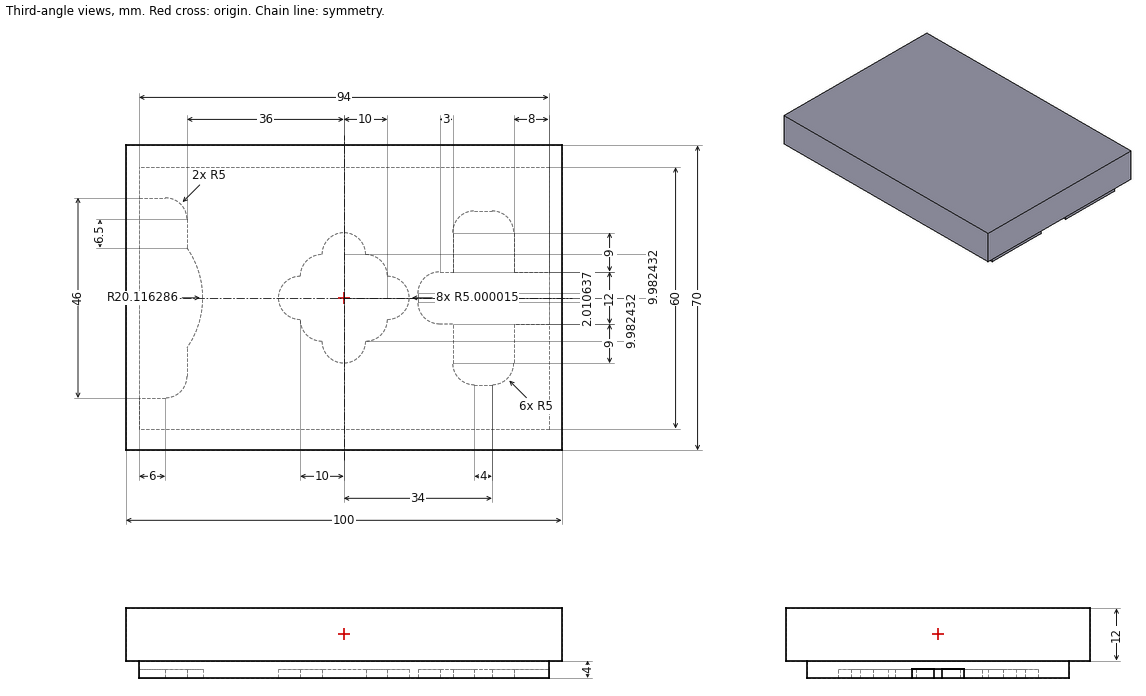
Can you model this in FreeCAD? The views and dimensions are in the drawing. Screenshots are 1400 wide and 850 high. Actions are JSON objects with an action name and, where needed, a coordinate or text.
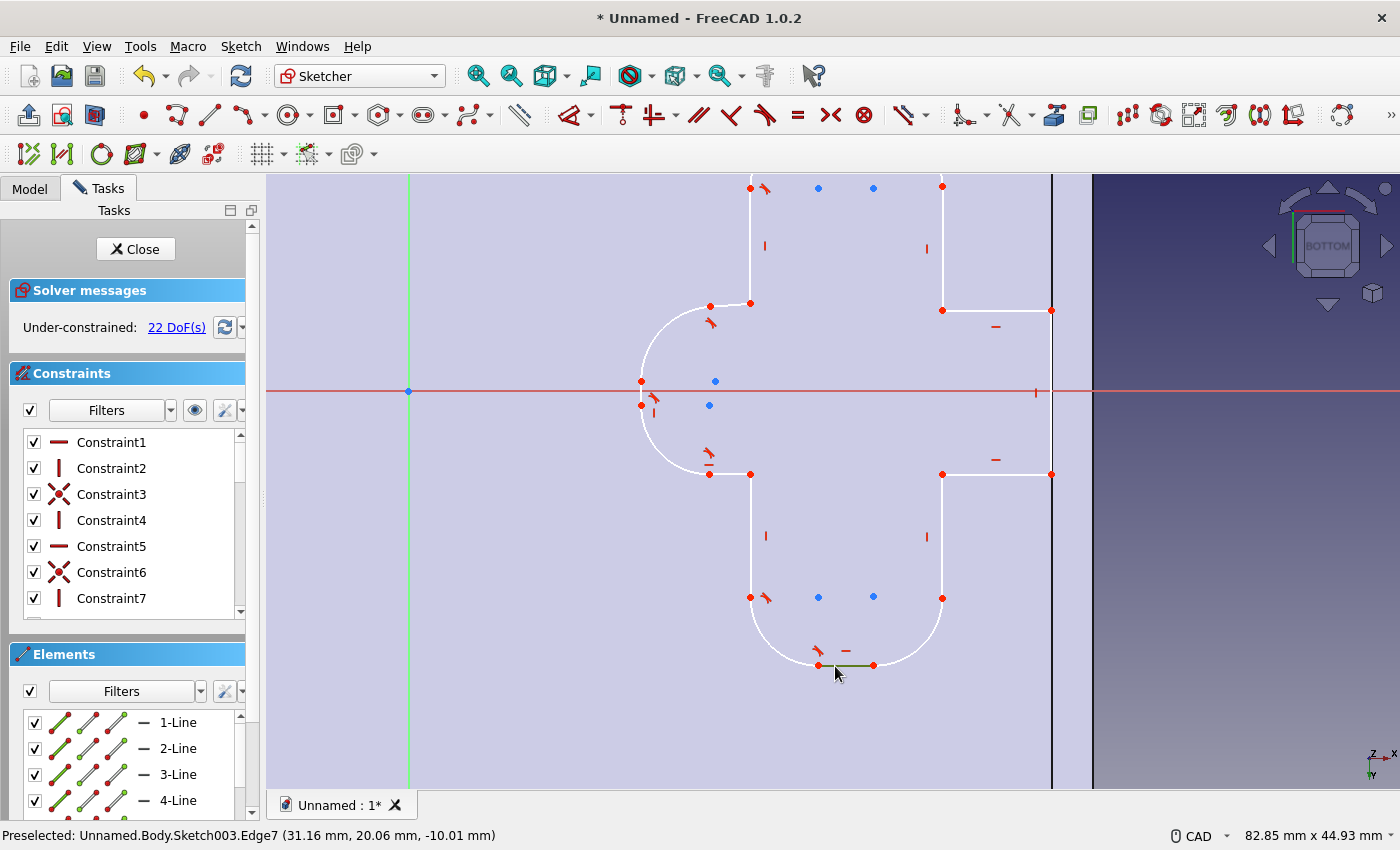
{"action": "left_click", "coordinate": [905, 658]}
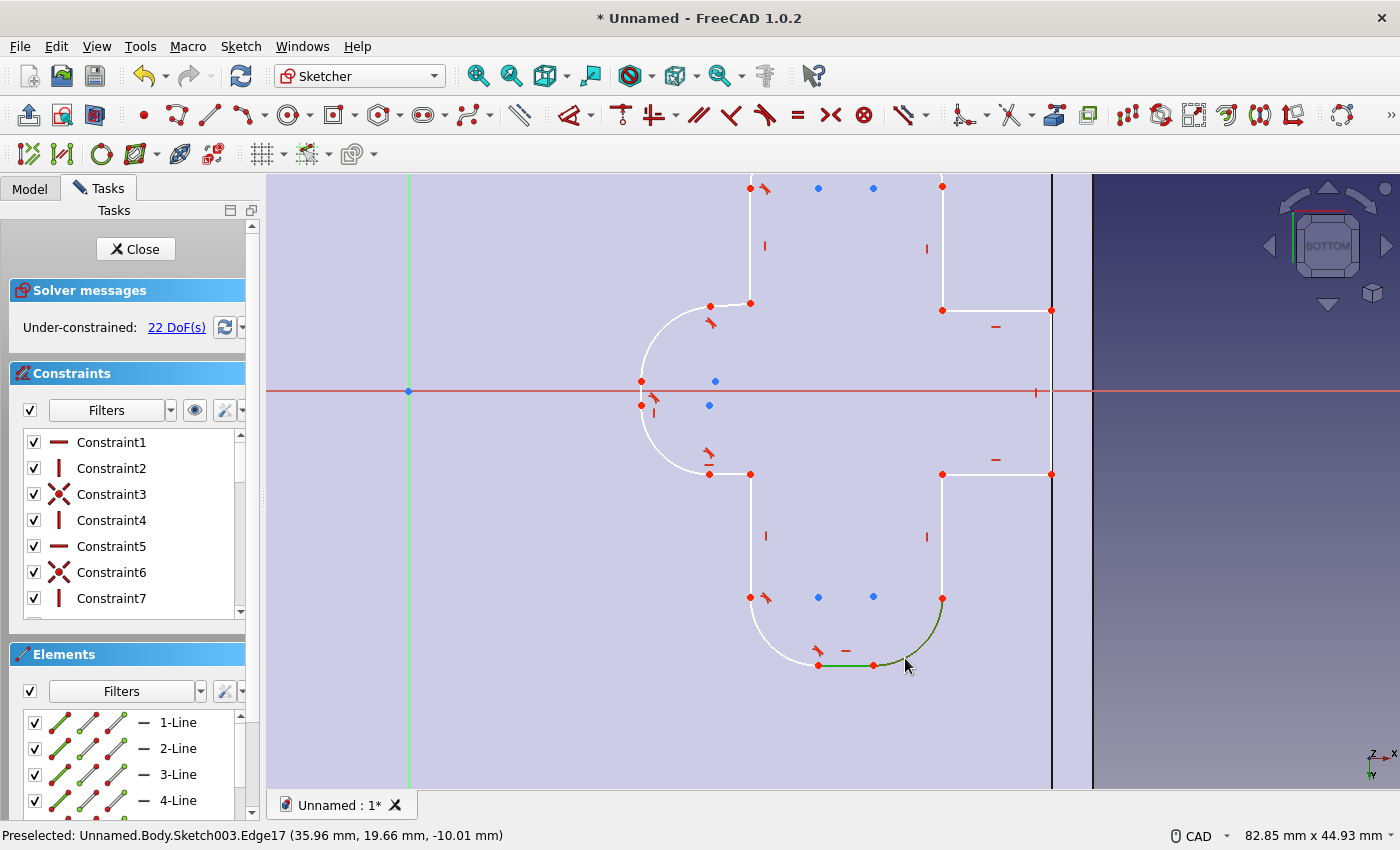
{"action": "left_click", "coordinate": [765, 116]}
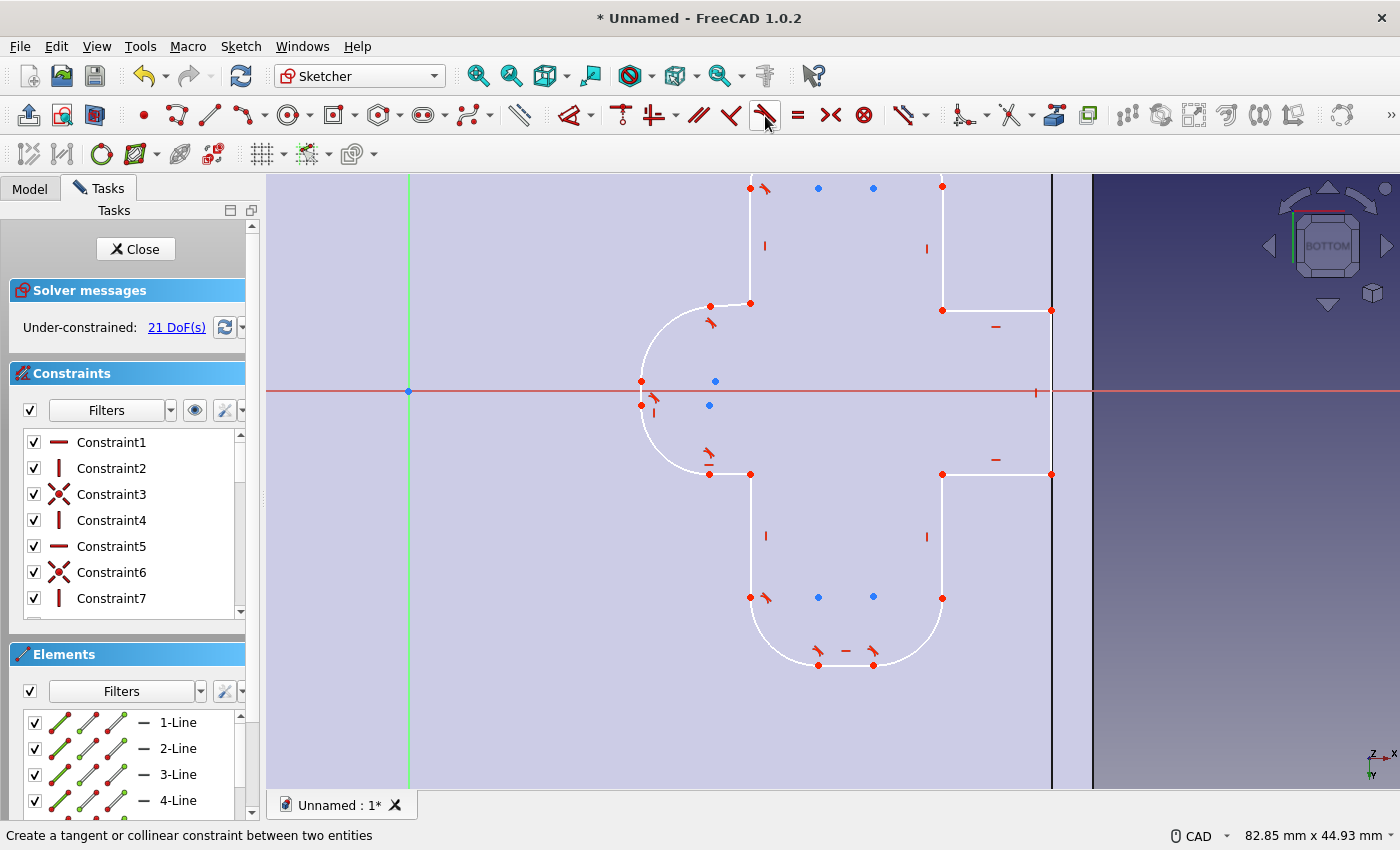
{"action": "left_click", "coordinate": [942, 561]}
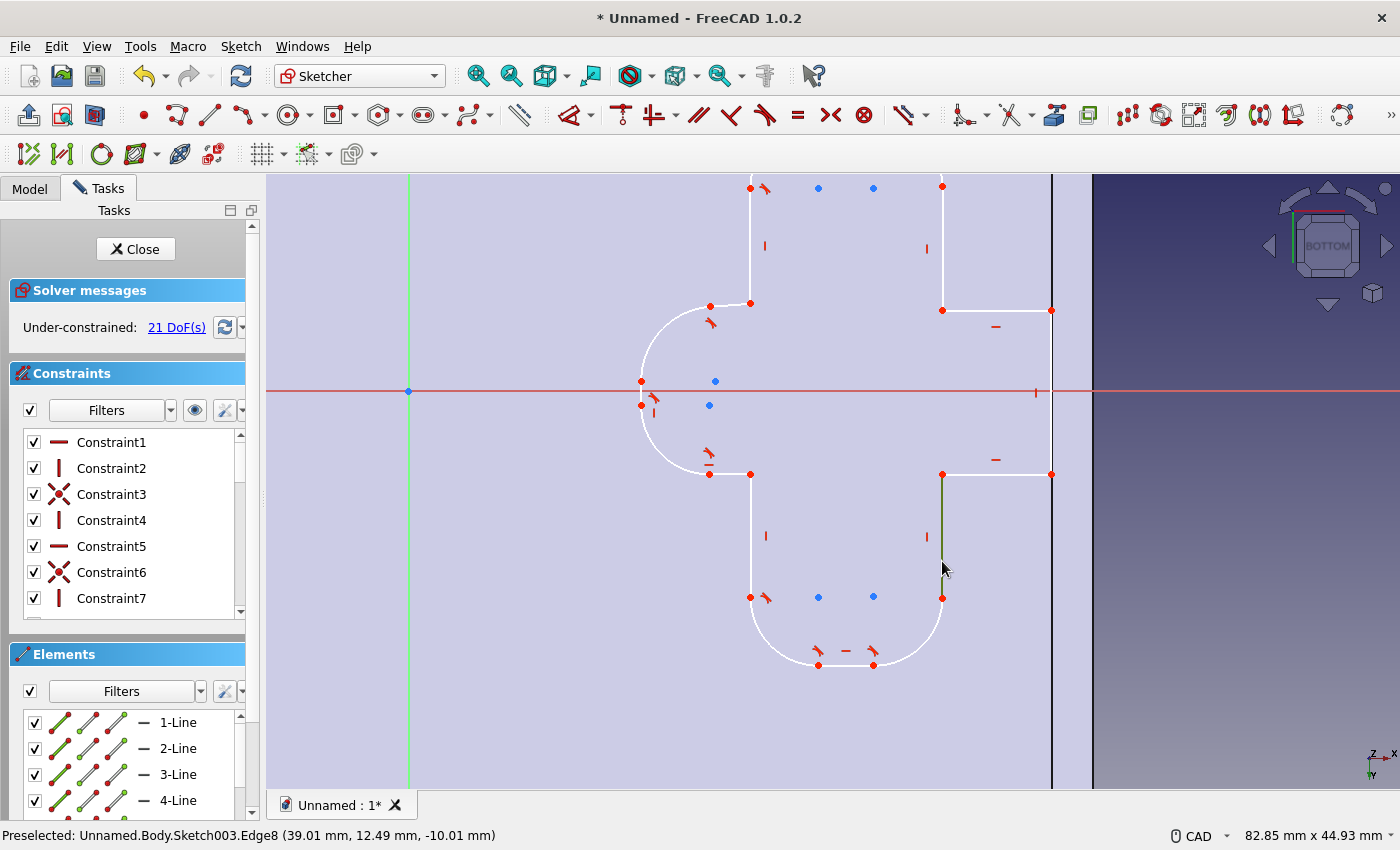
{"action": "left_click", "coordinate": [905, 658]}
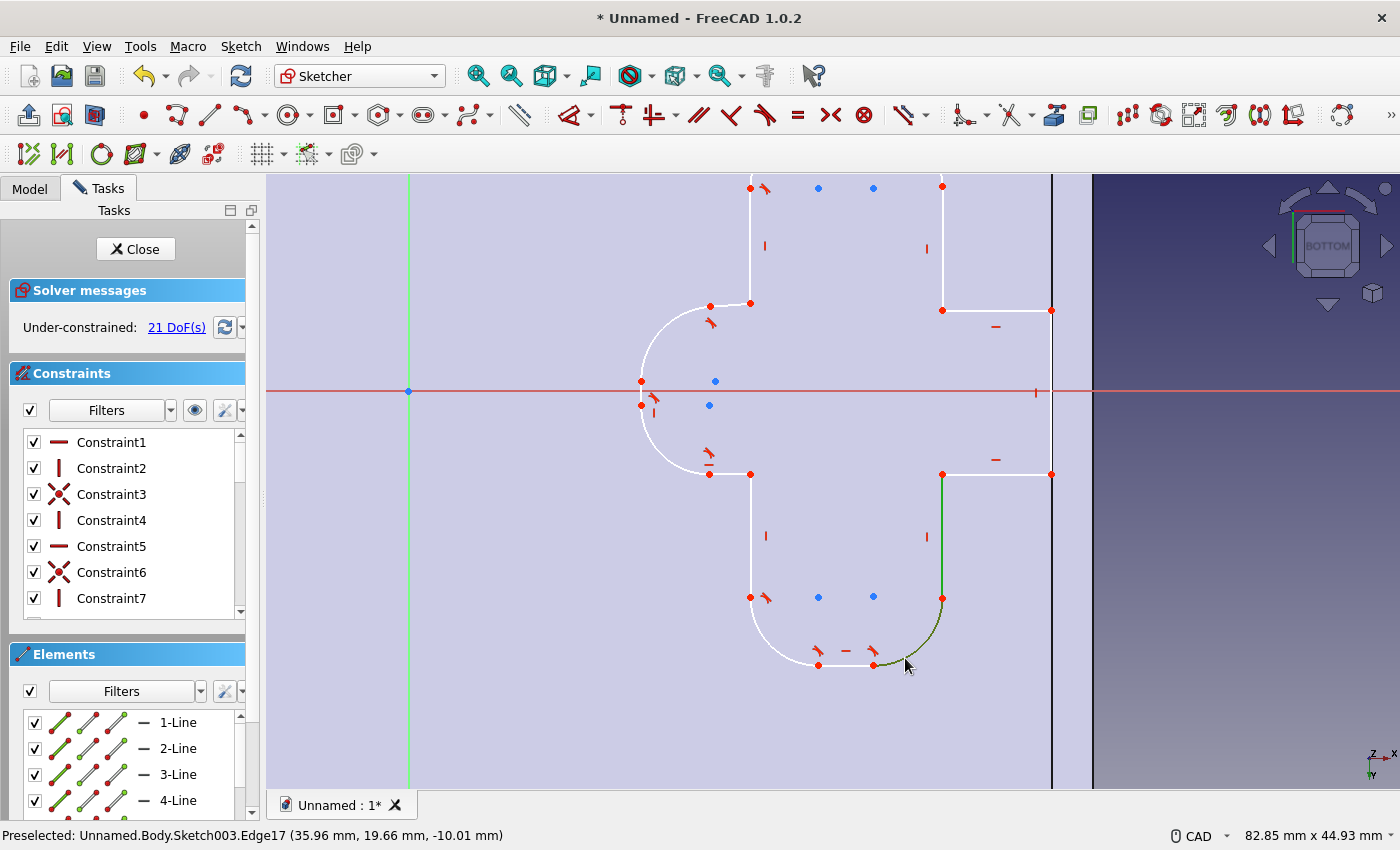
{"action": "left_click", "coordinate": [765, 116]}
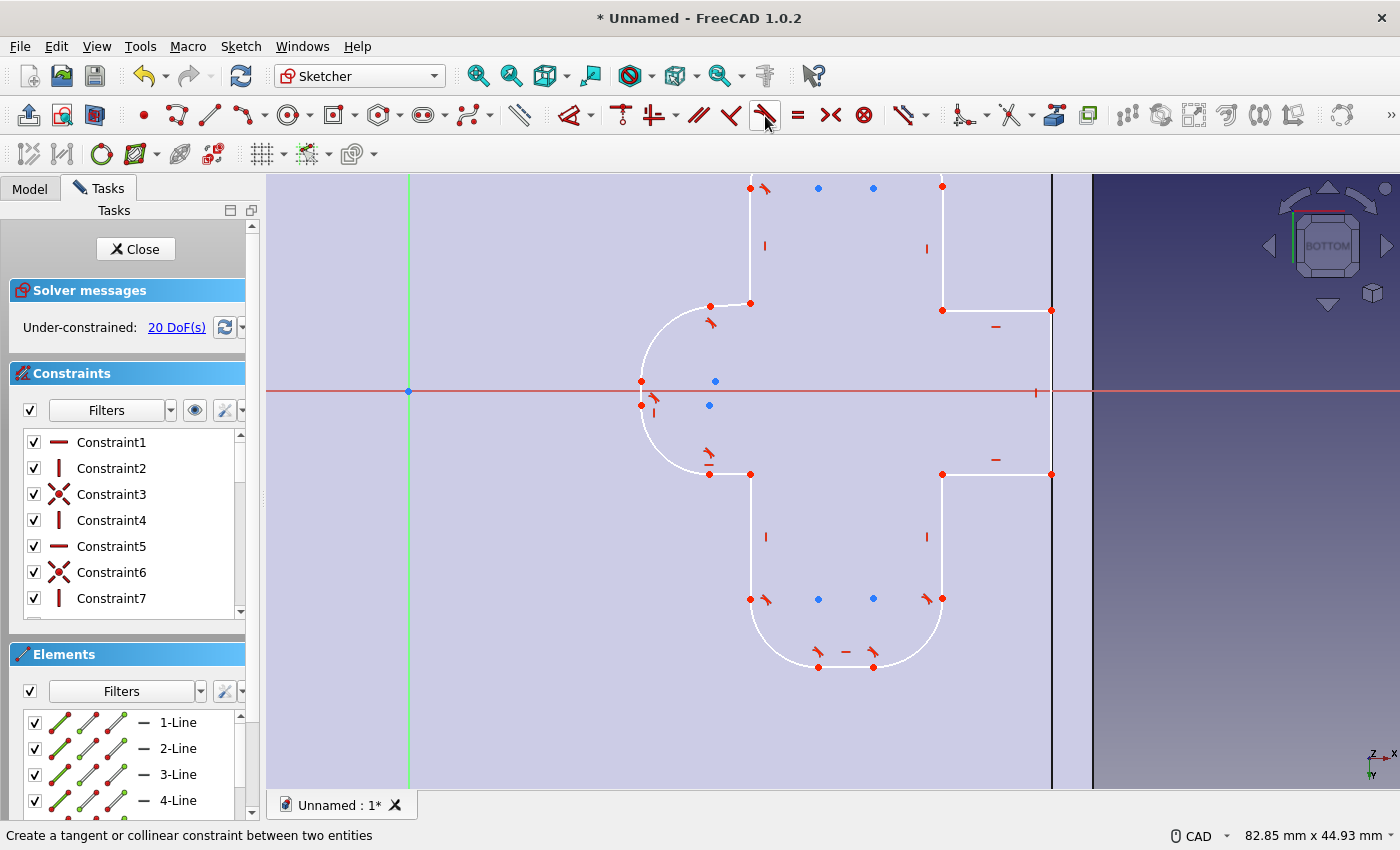
{"action": "left_click", "coordinate": [943, 274]}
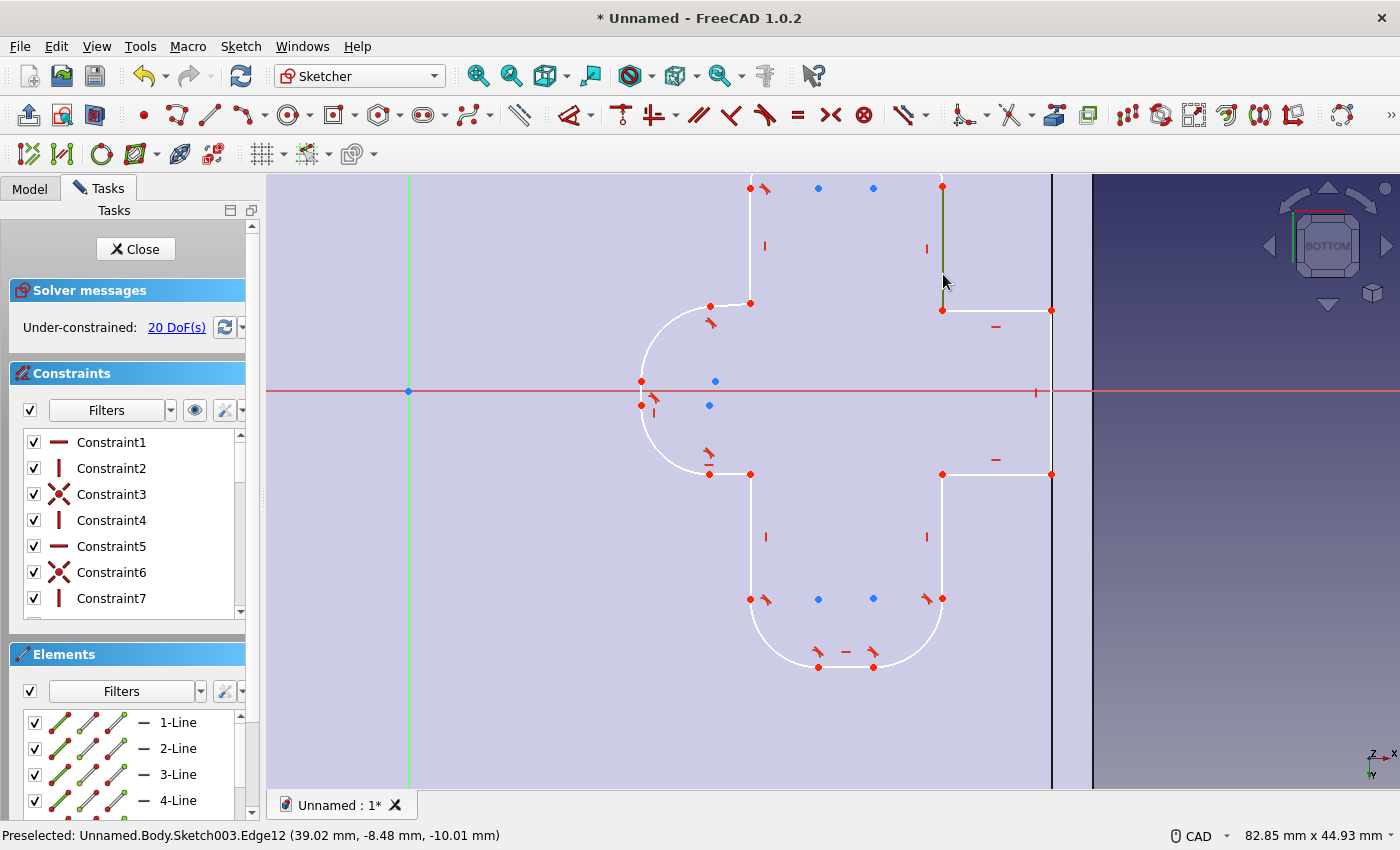
{"action": "scroll", "coordinate": [834, 665], "scroll_direction": "down", "scroll_amount": 2}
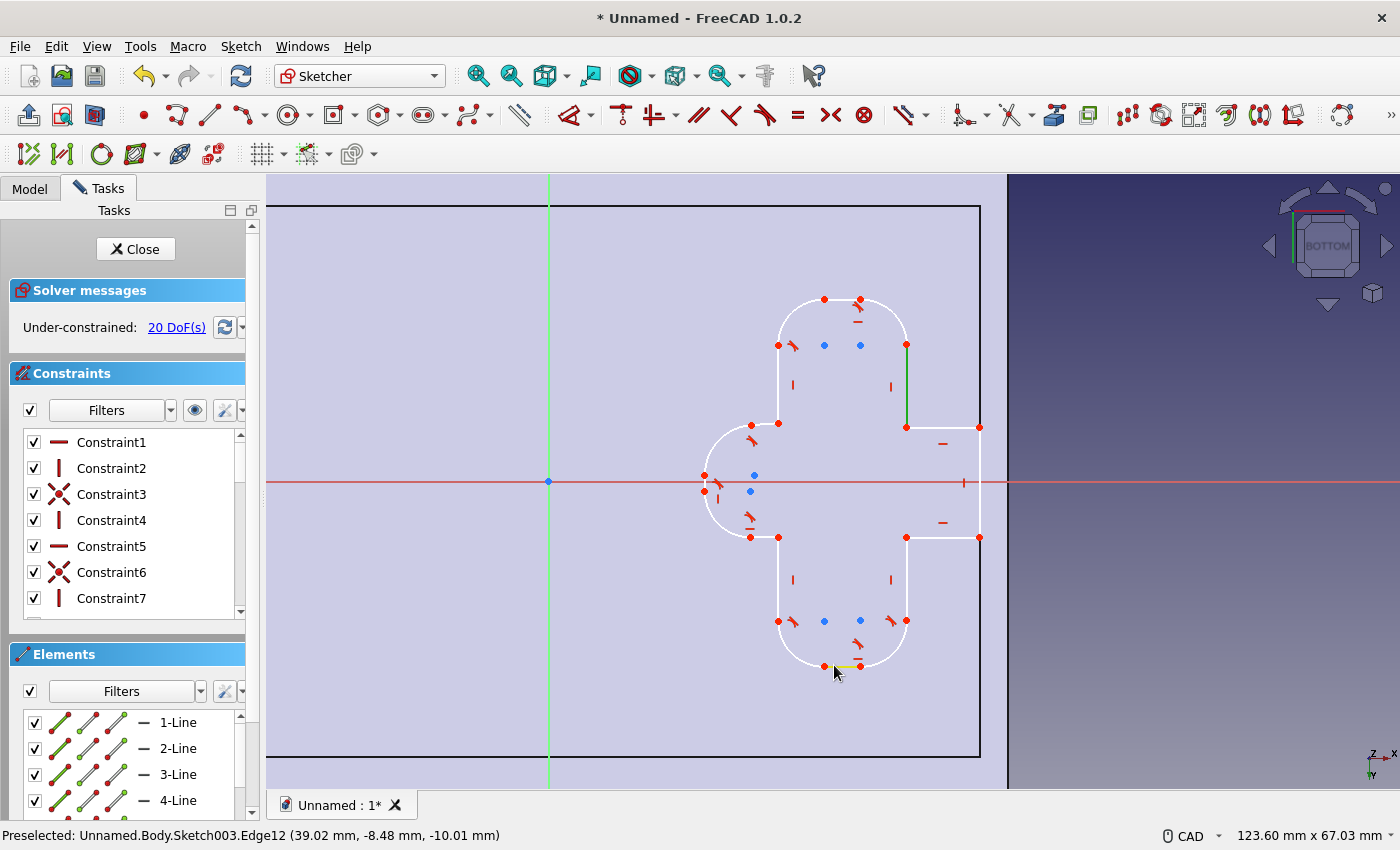
{"action": "left_click", "coordinate": [902, 324]}